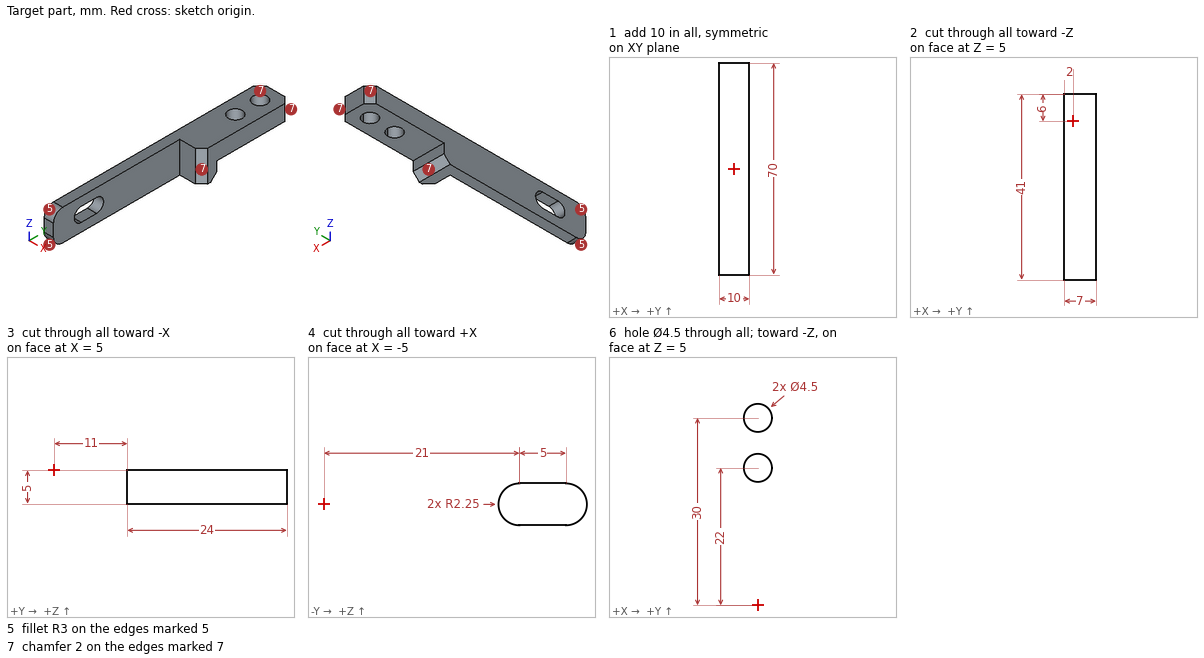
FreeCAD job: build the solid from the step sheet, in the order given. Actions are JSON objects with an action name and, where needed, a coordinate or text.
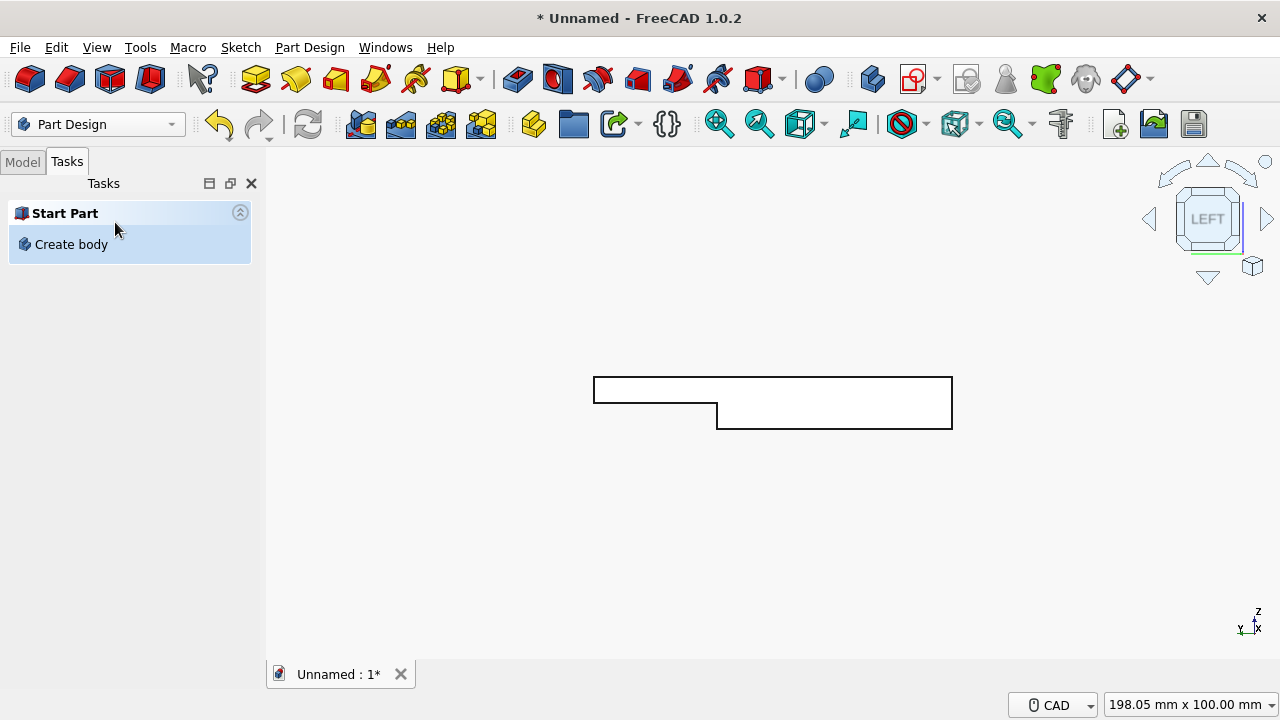
{"action": "key", "text": "v f"}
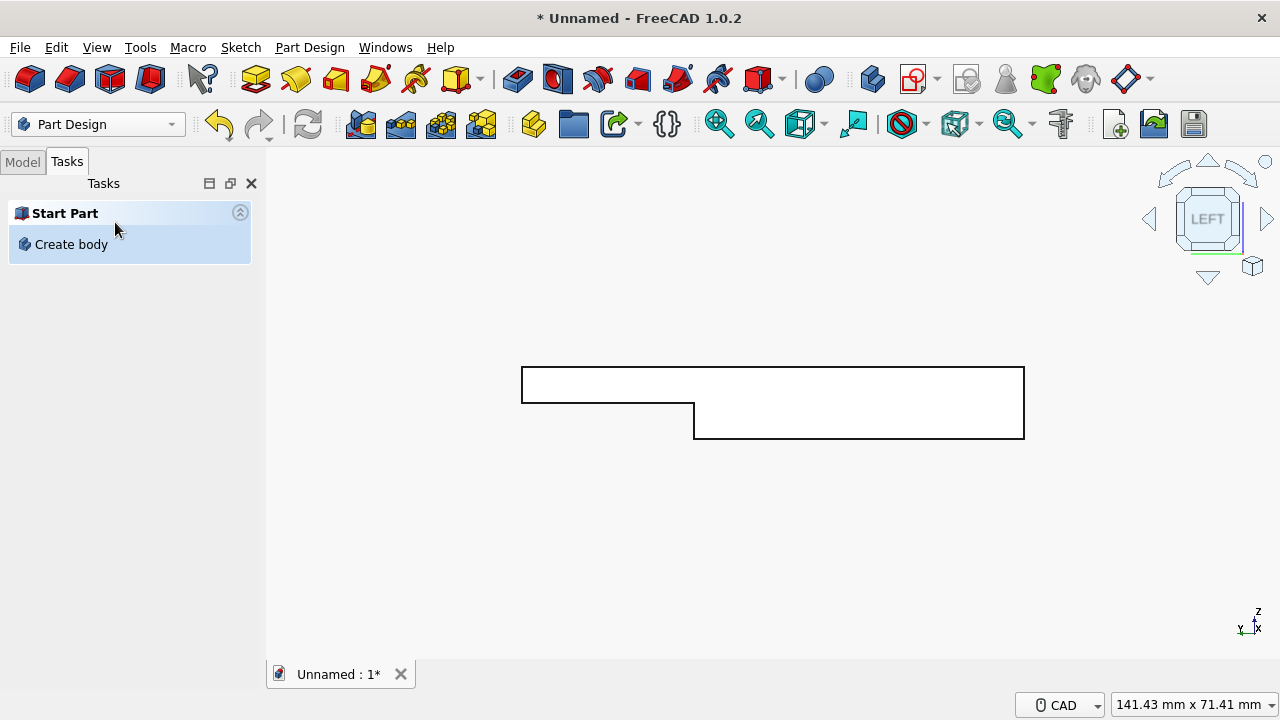
{"action": "left_click", "coordinate": [773, 402]}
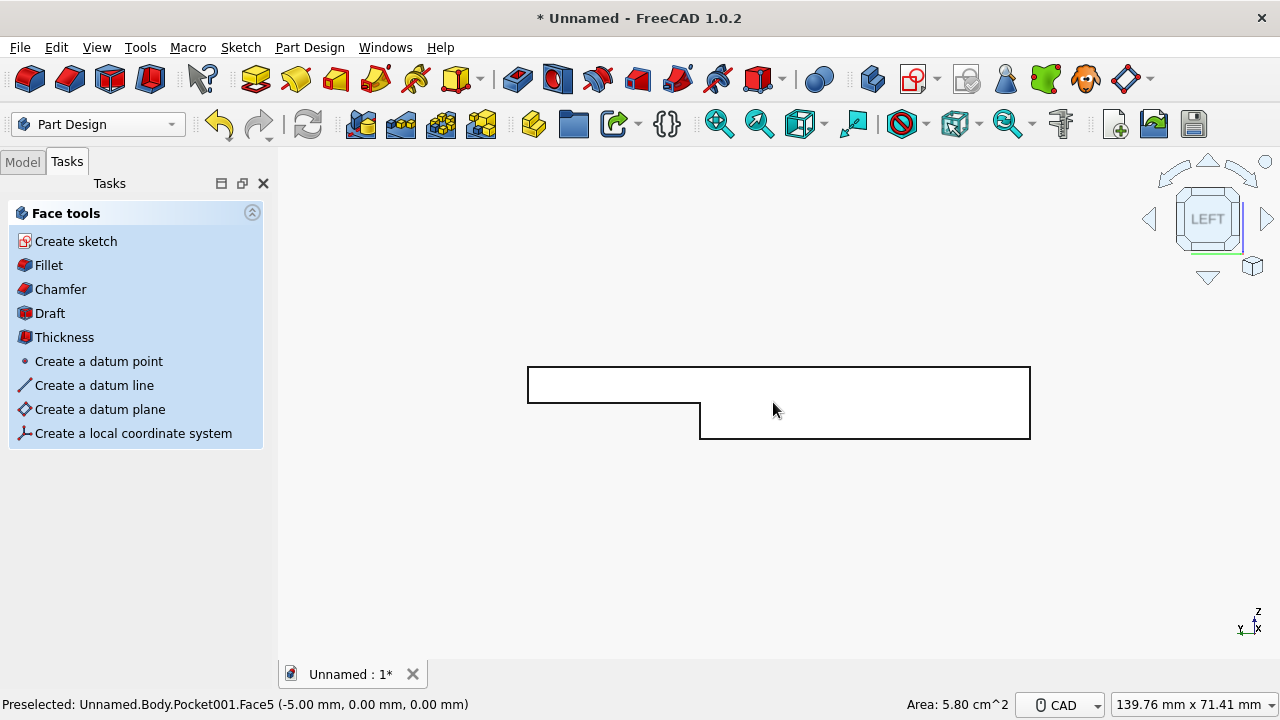
{"action": "left_click", "coordinate": [914, 80]}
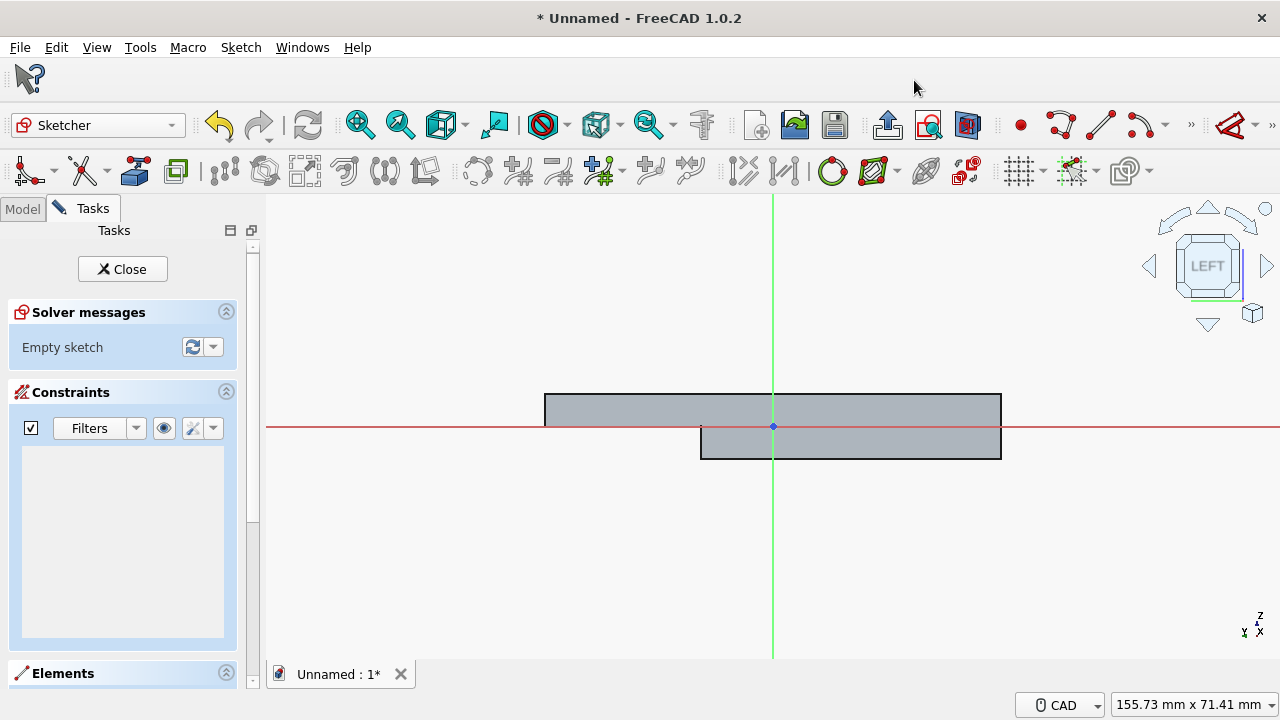
{"action": "scroll", "coordinate": [954, 426], "scroll_direction": "up", "scroll_amount": 11}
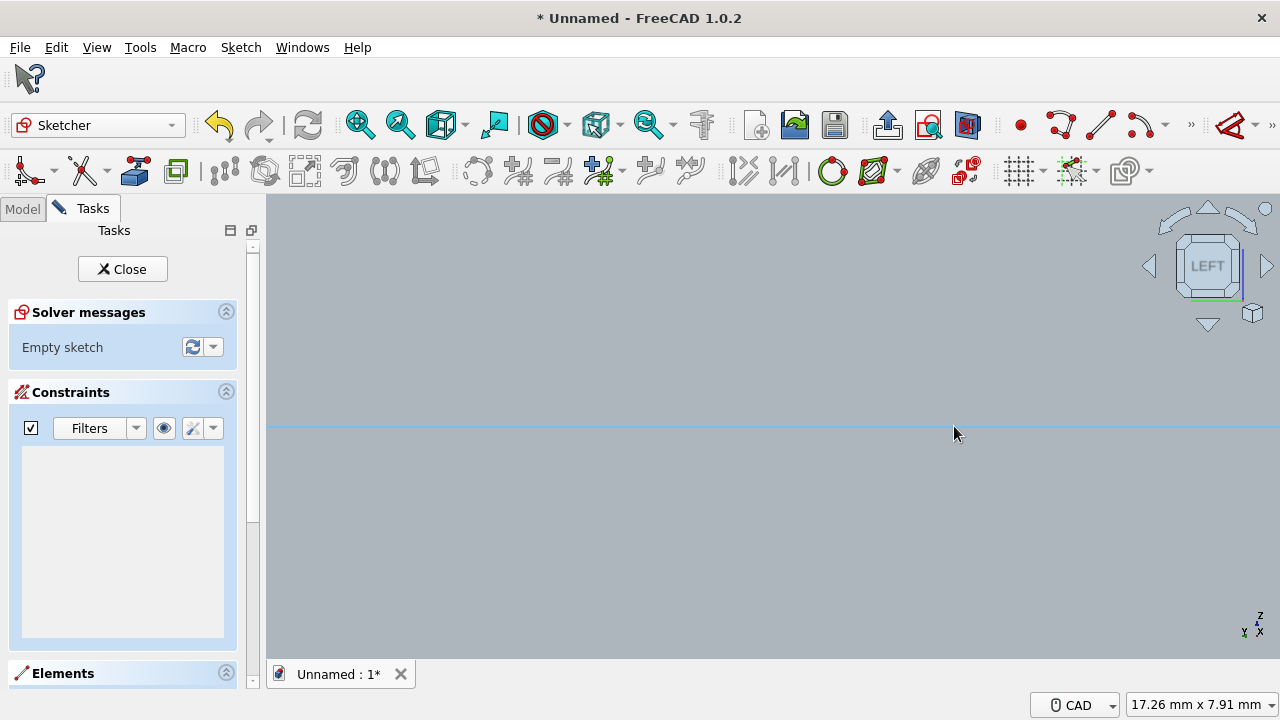
{"action": "key", "text": "g s"}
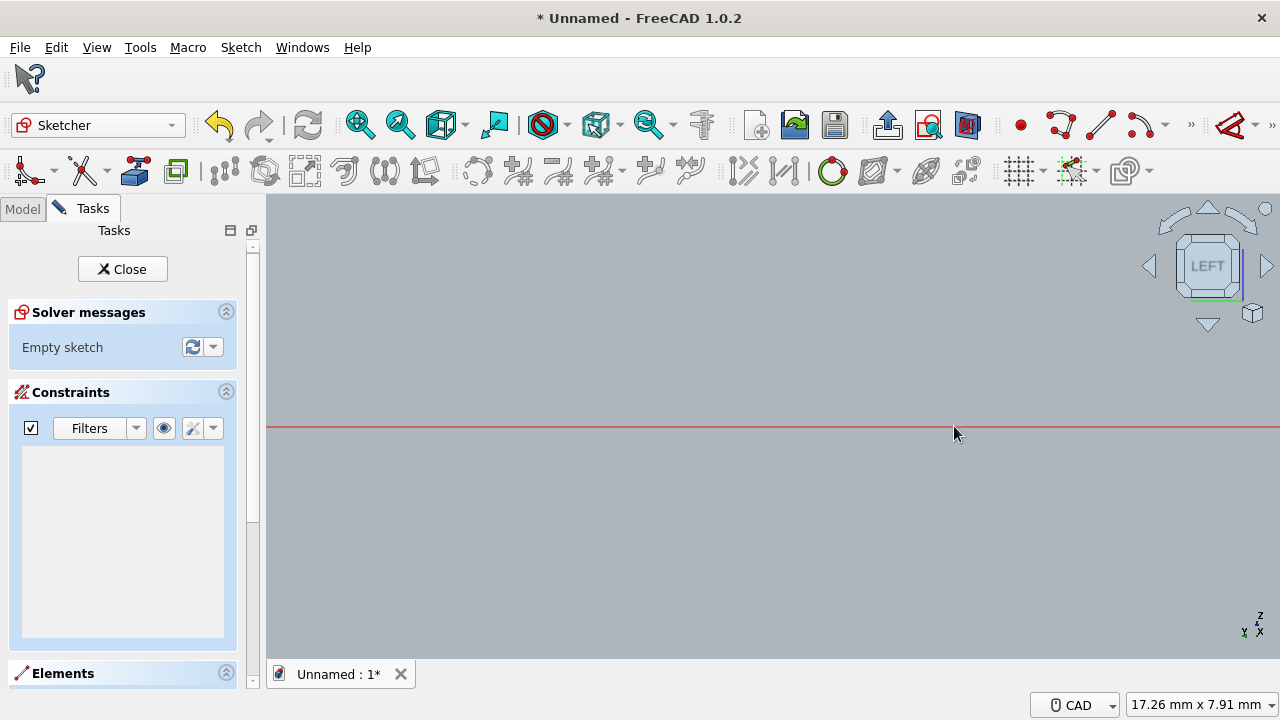
{"action": "left_click", "coordinate": [549, 426]}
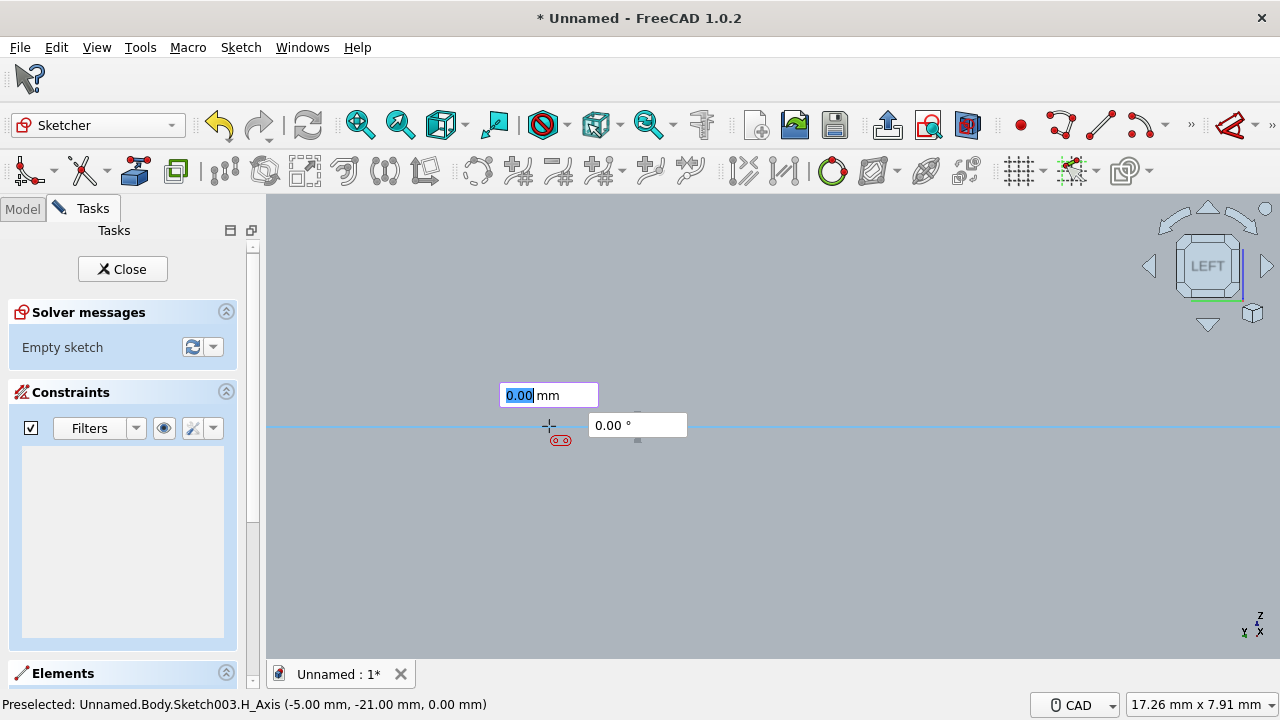
{"action": "left_click", "coordinate": [843, 418]}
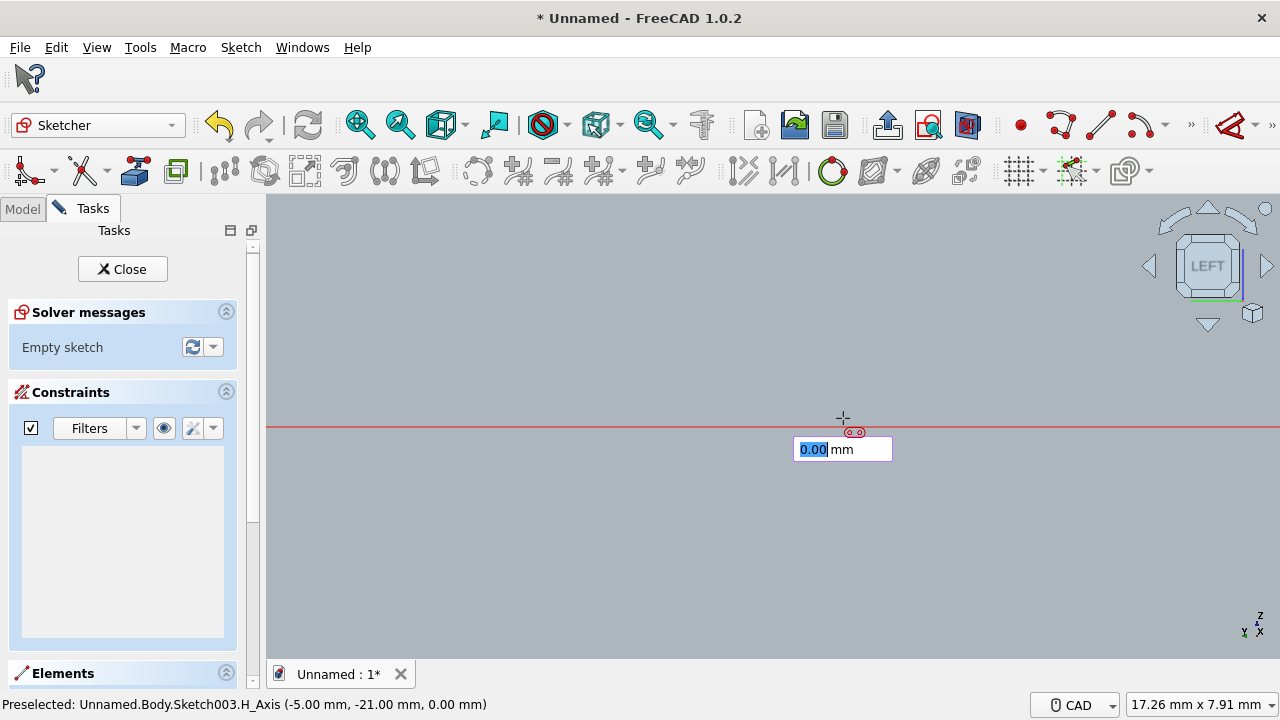
{"action": "left_click", "coordinate": [696, 294]}
{"action": "key", "text": "Escape"}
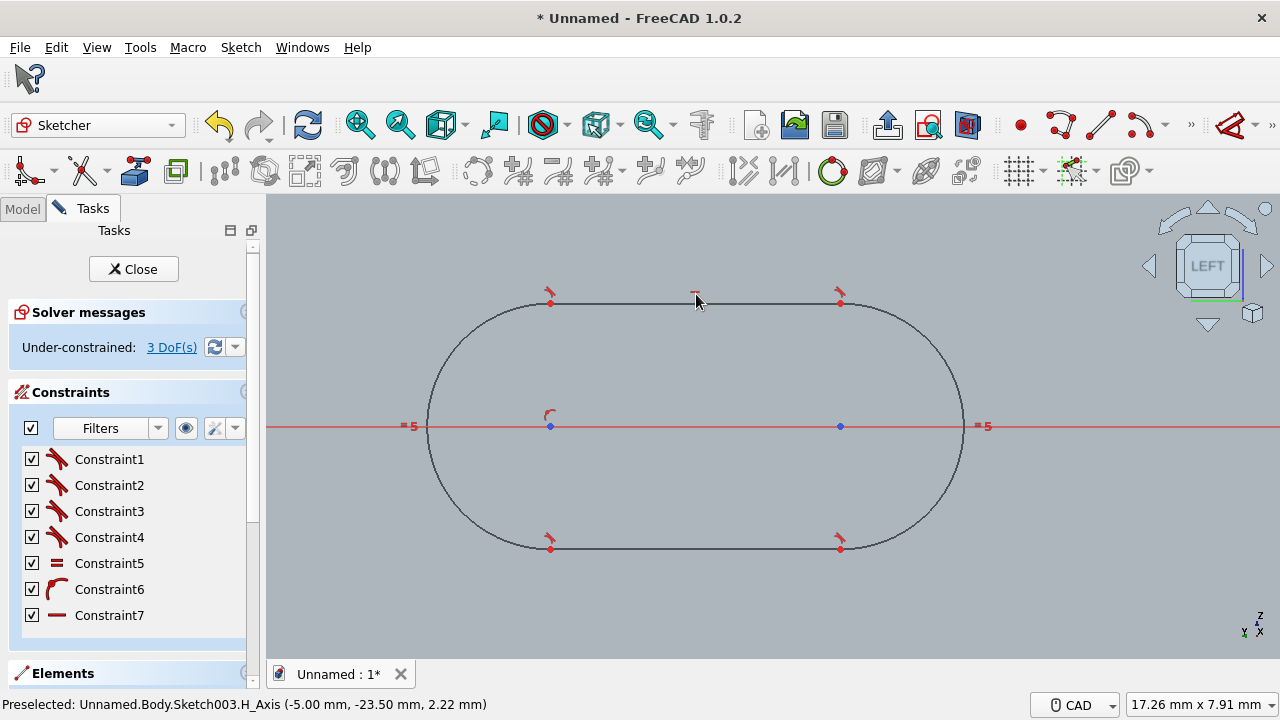
{"action": "left_click", "coordinate": [1230, 126]}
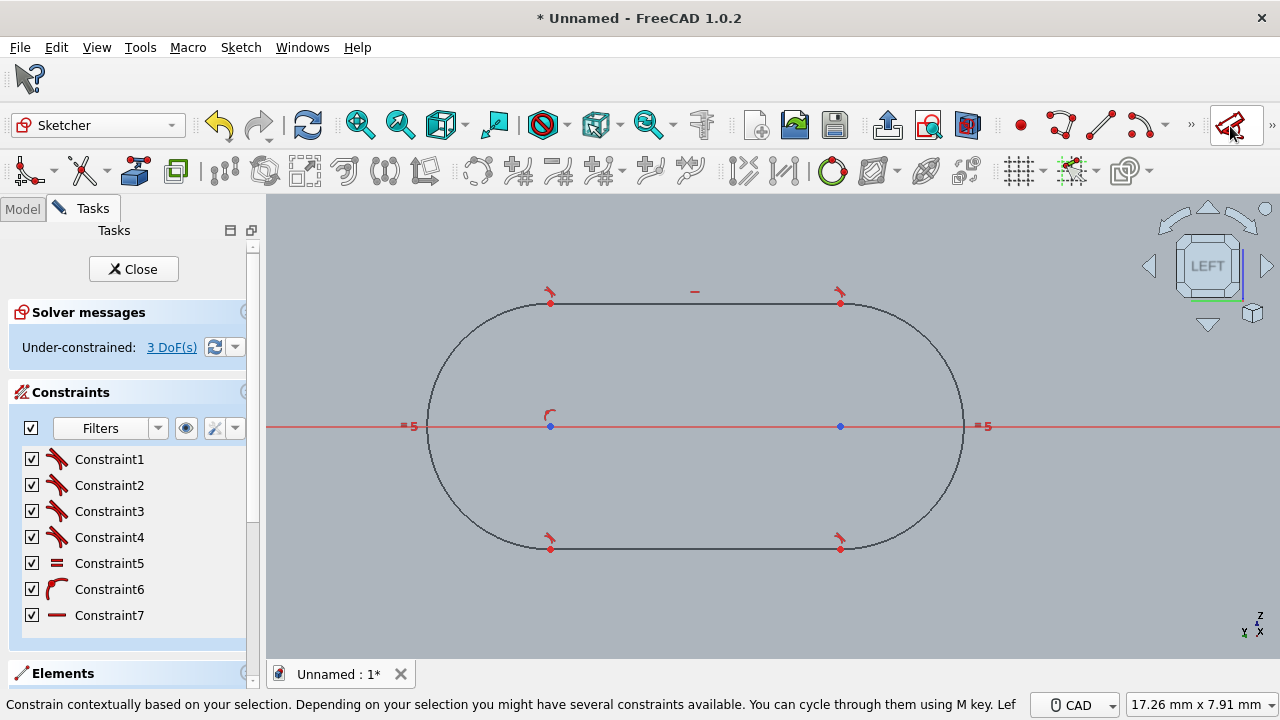
{"action": "left_click", "coordinate": [451, 354]}
{"action": "left_click", "coordinate": [425, 335]}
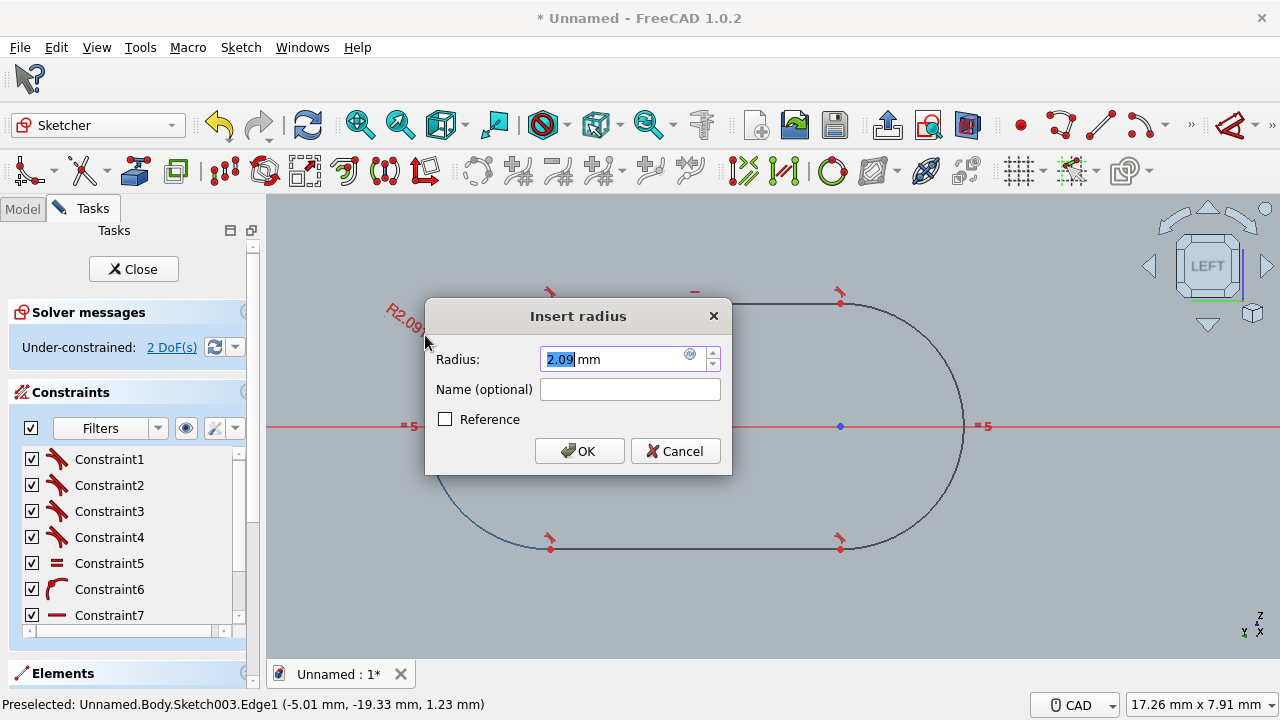
{"action": "type", "text": "2.25"}
{"action": "key", "text": "Return"}